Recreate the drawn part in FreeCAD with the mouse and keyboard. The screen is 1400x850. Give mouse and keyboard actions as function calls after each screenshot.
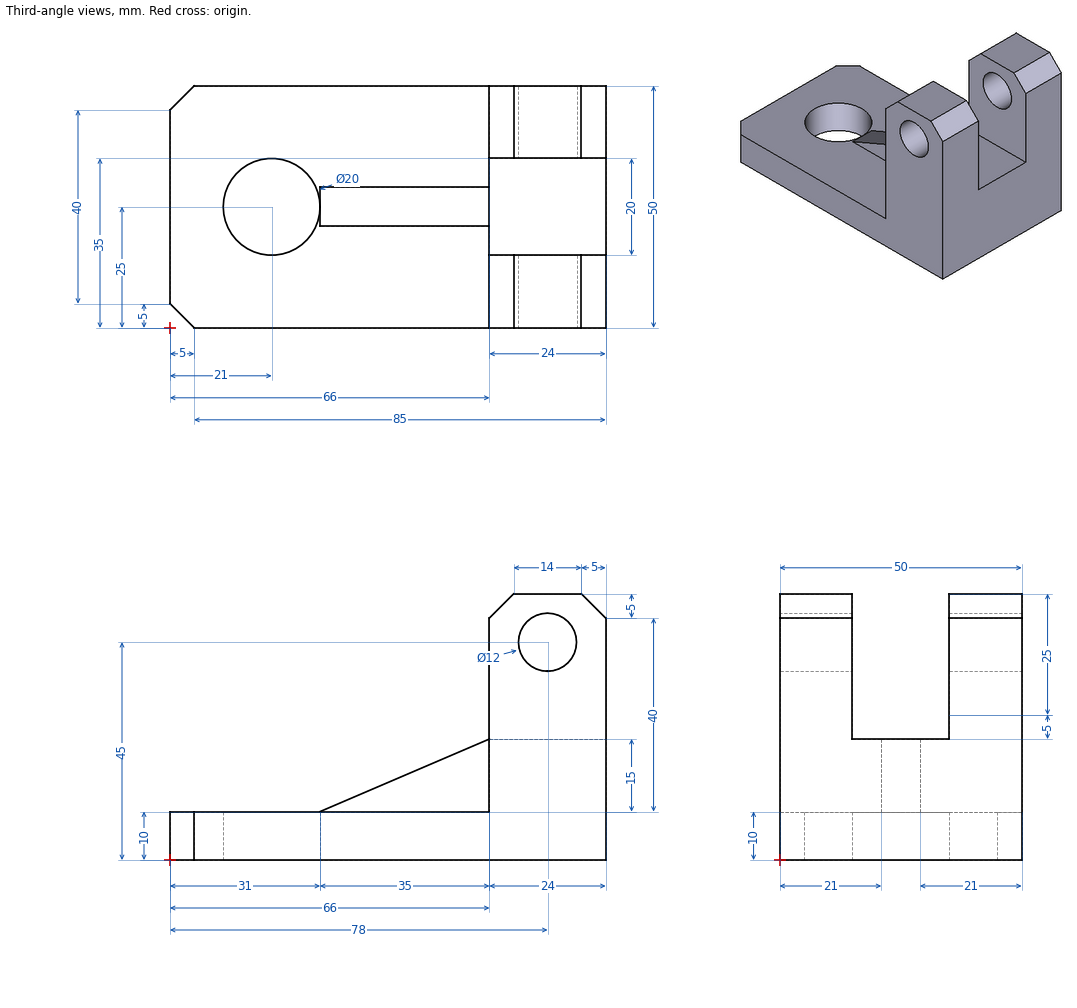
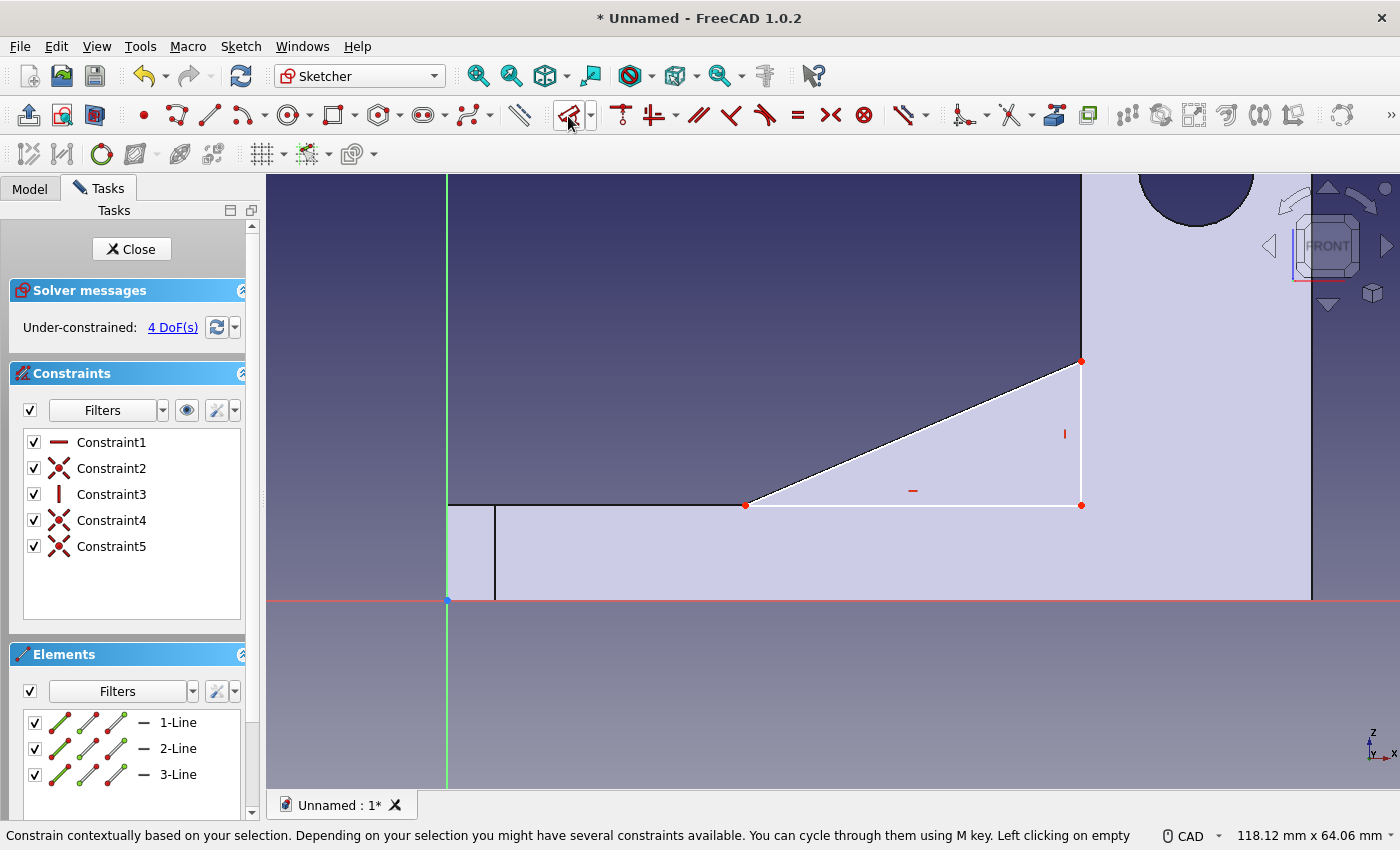
click(846, 506)
click(913, 540)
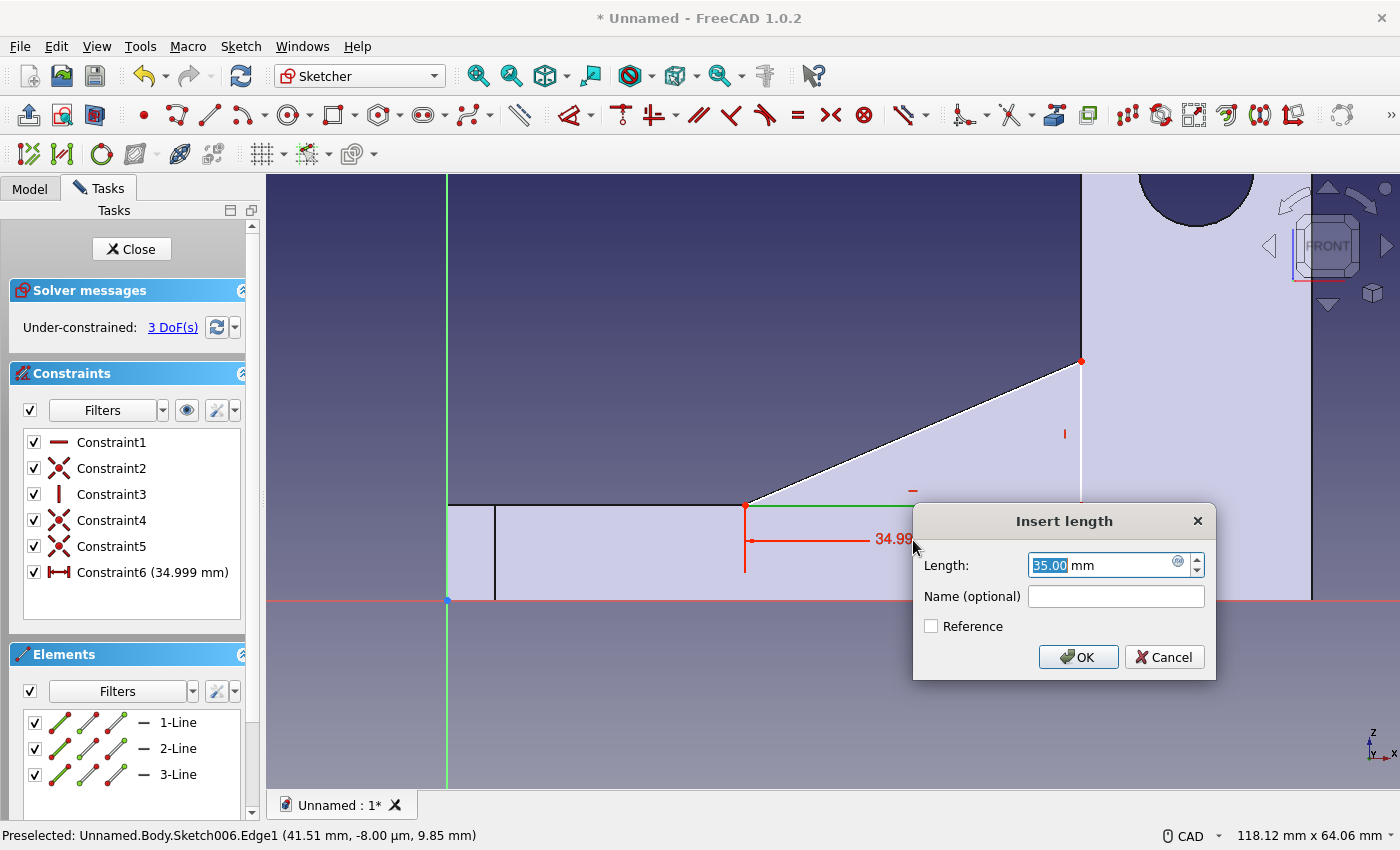
text(35)
key(Return)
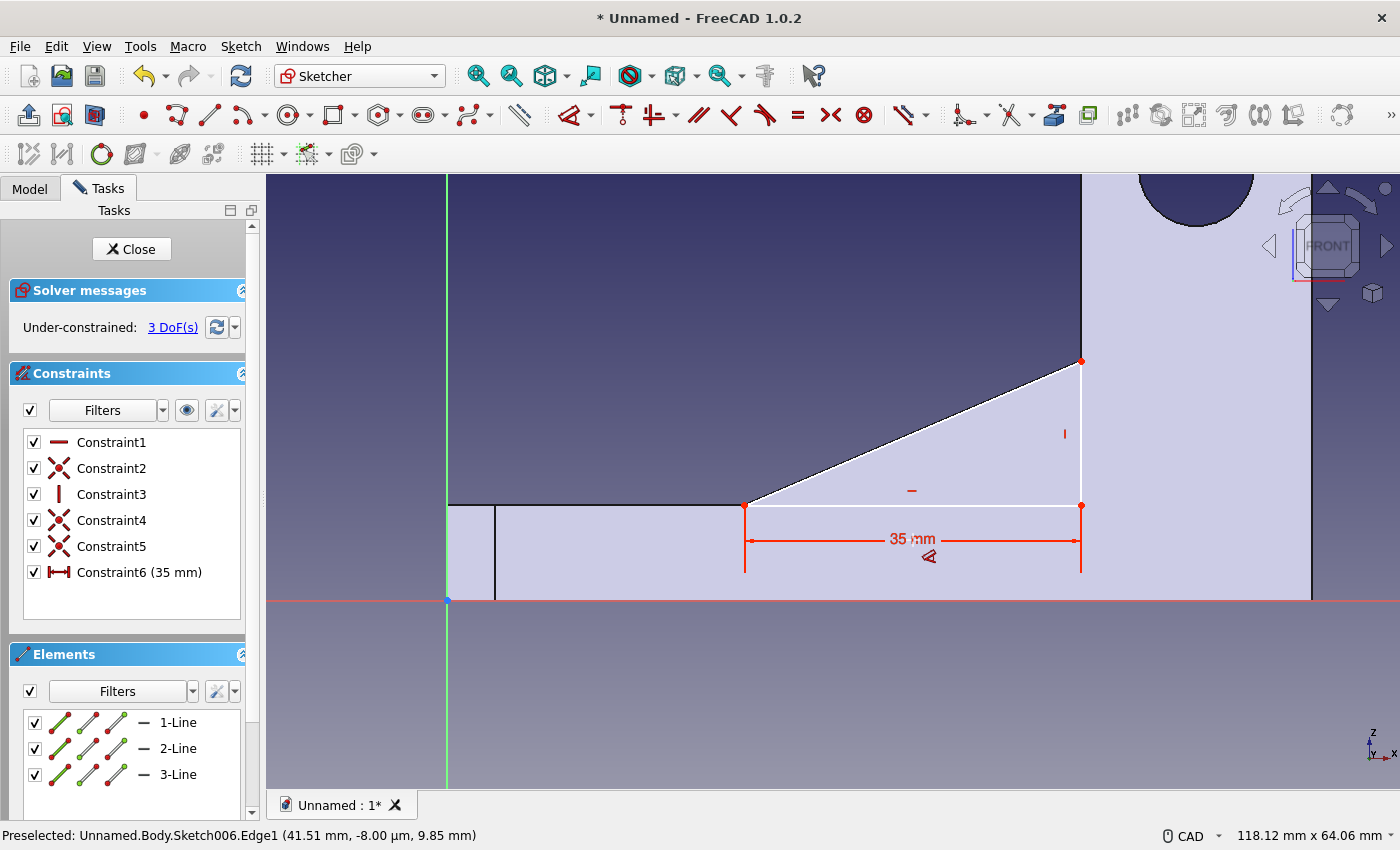
click(1081, 463)
click(1115, 434)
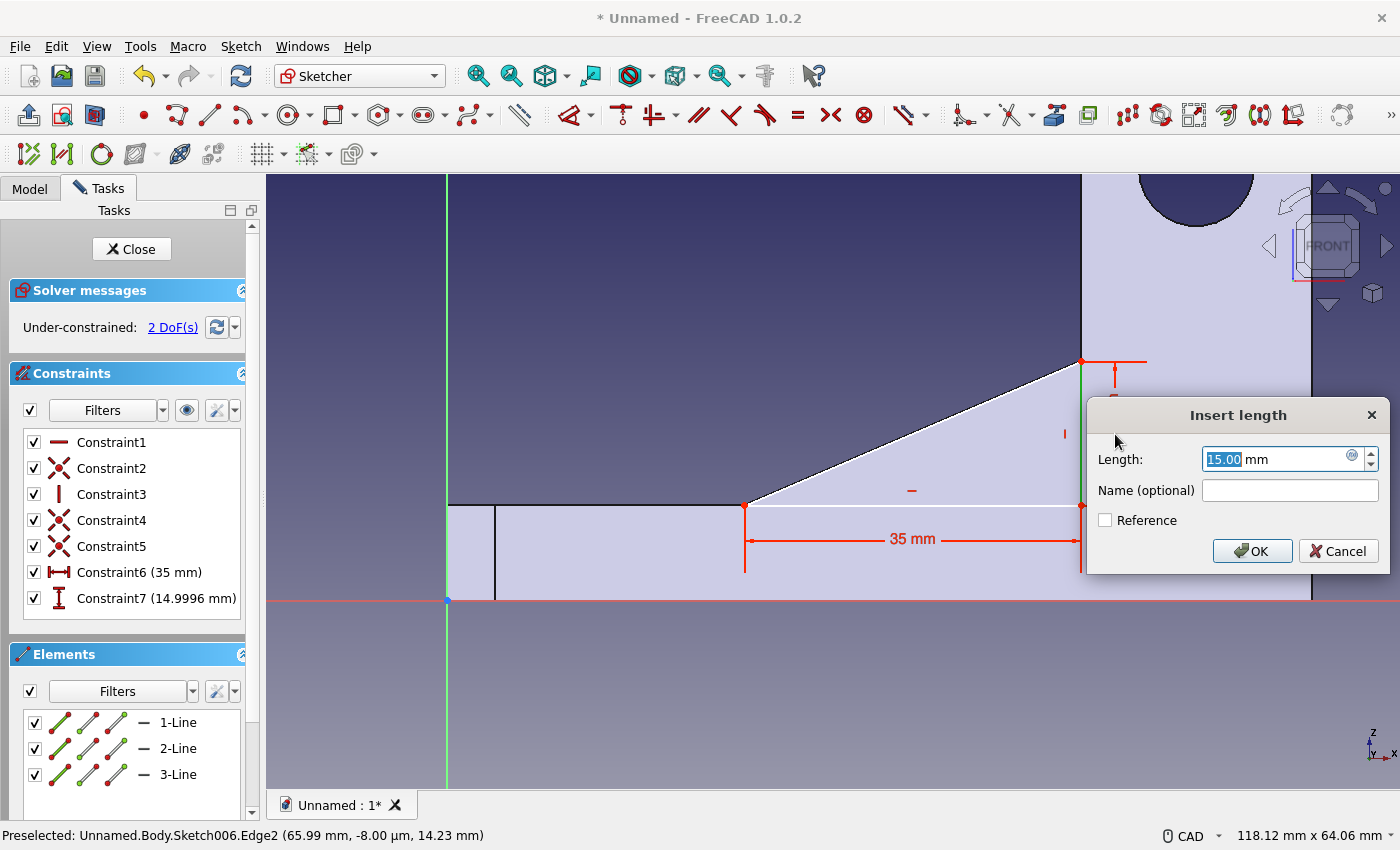
text(15)
key(Return)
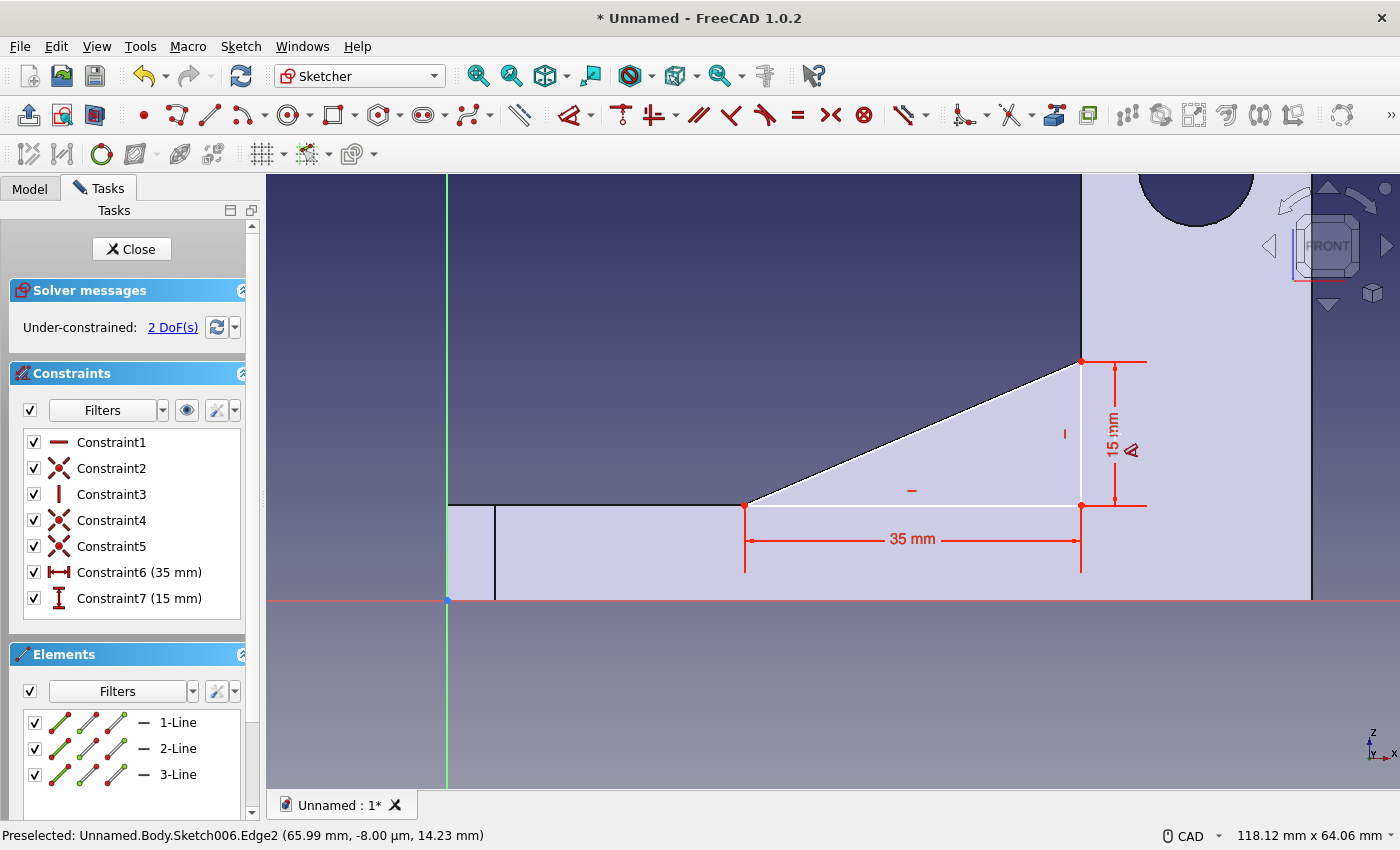
click(745, 506)
click(596, 635)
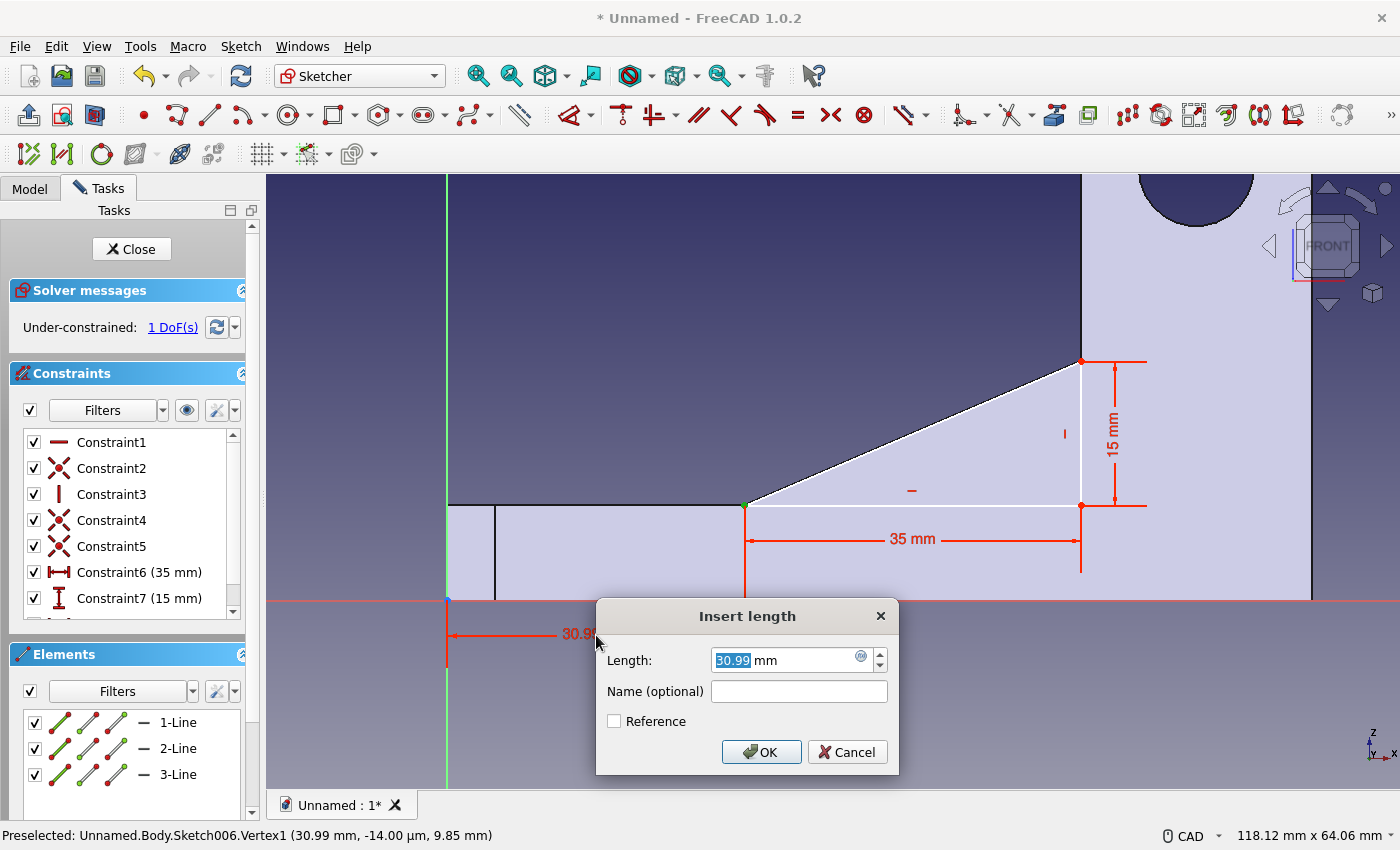
text(31)
key(Return)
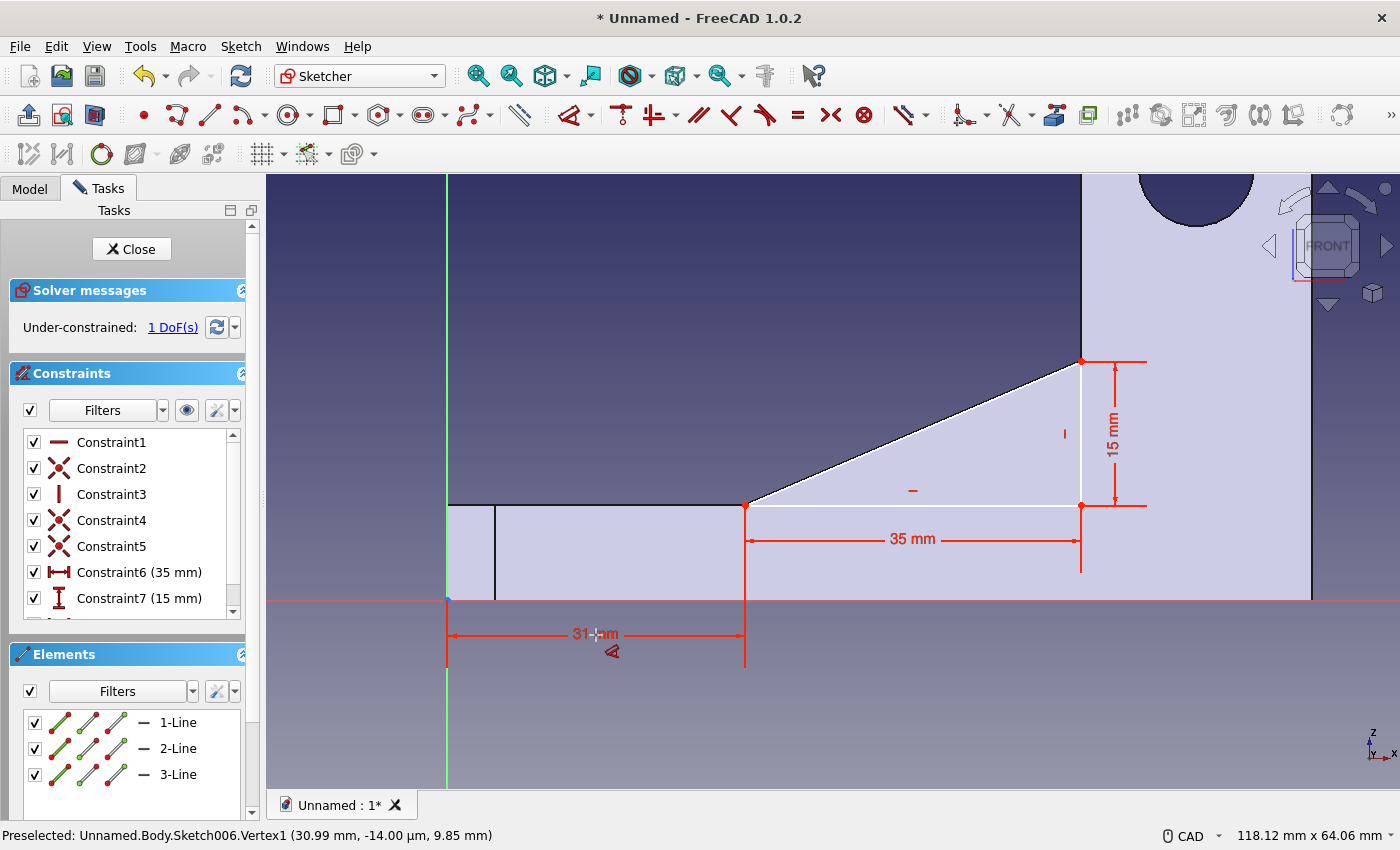
click(745, 506)
click(413, 553)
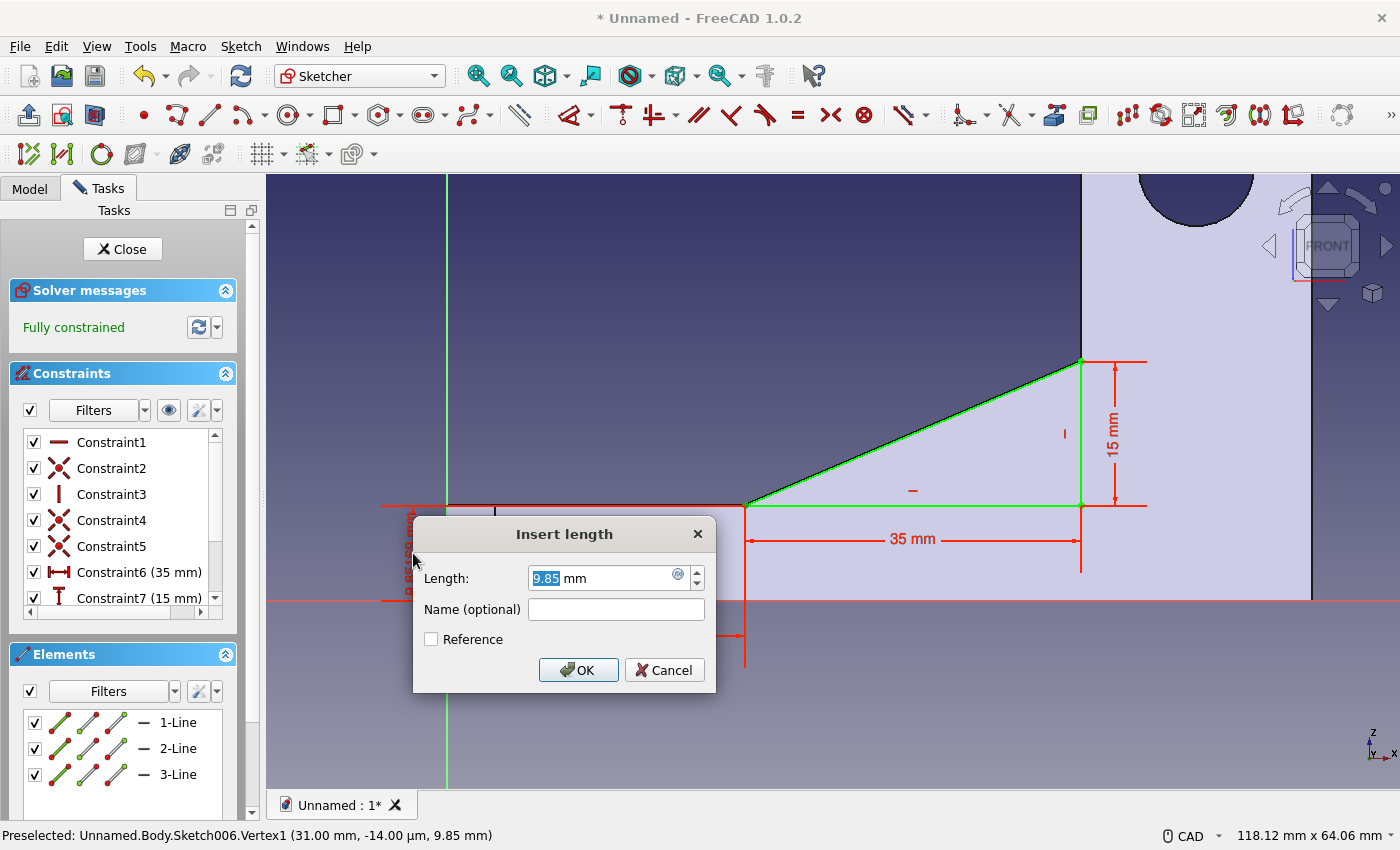
text(10)
key(Return)
key(Escape)